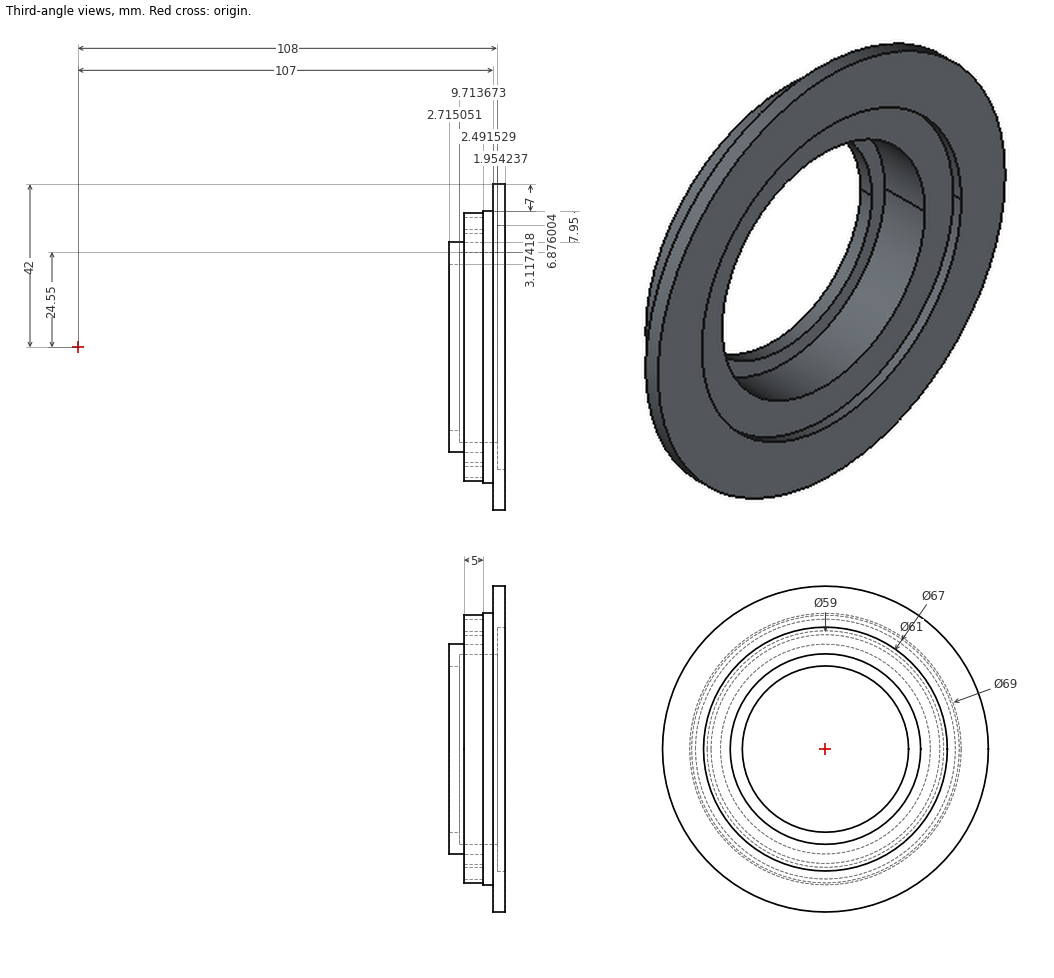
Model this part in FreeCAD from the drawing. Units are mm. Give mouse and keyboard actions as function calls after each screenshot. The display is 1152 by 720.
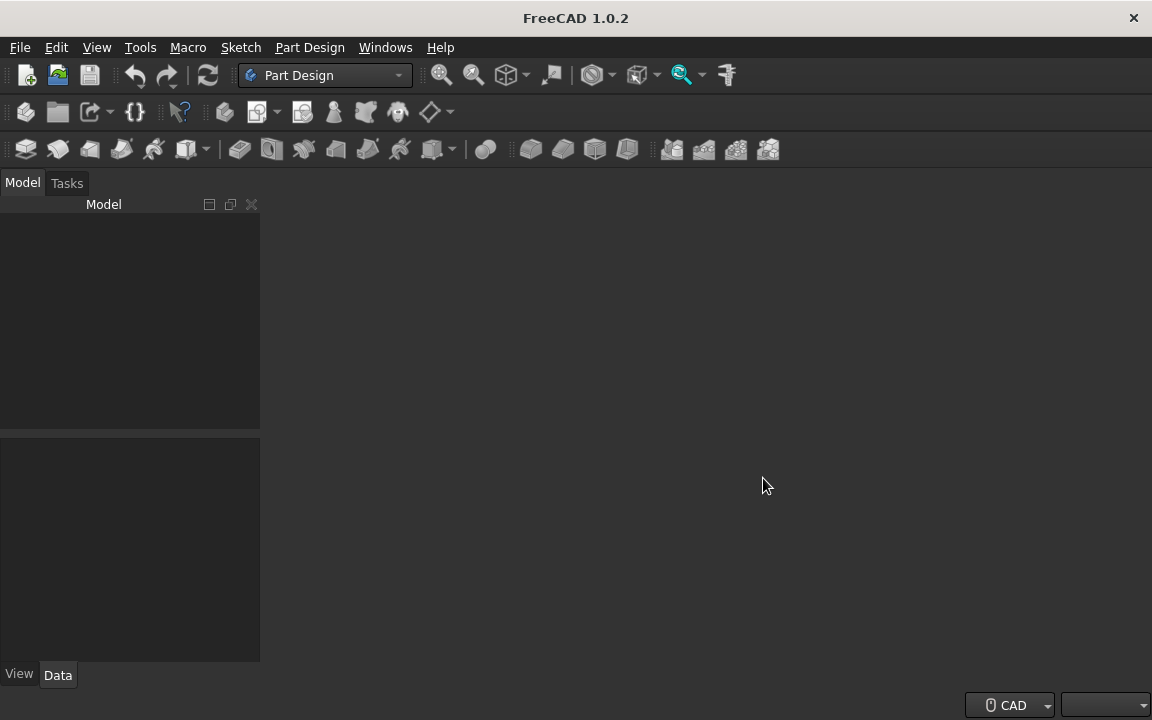
click(26, 76)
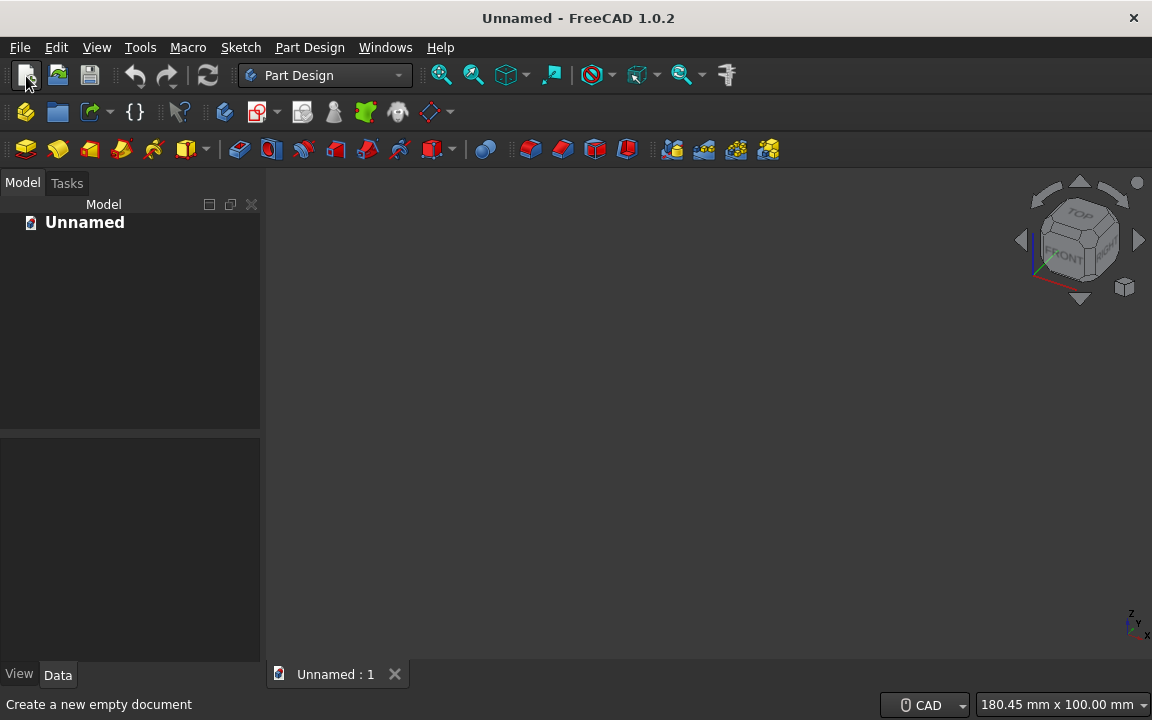
click(258, 112)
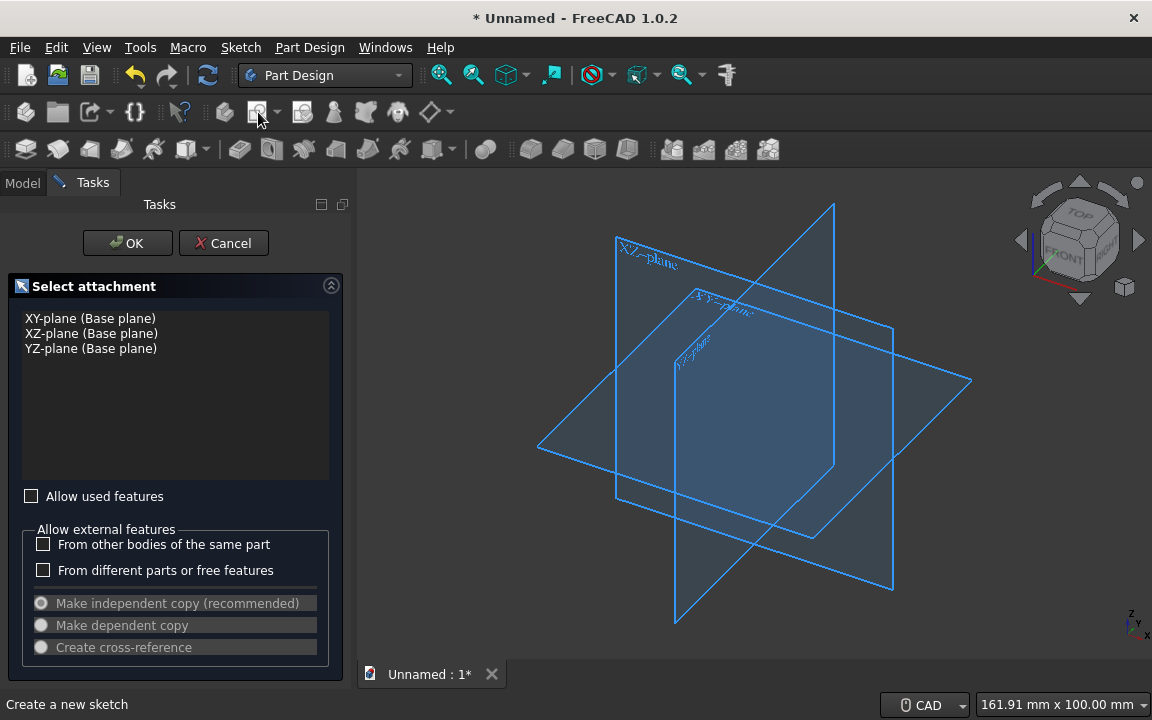
click(82, 318)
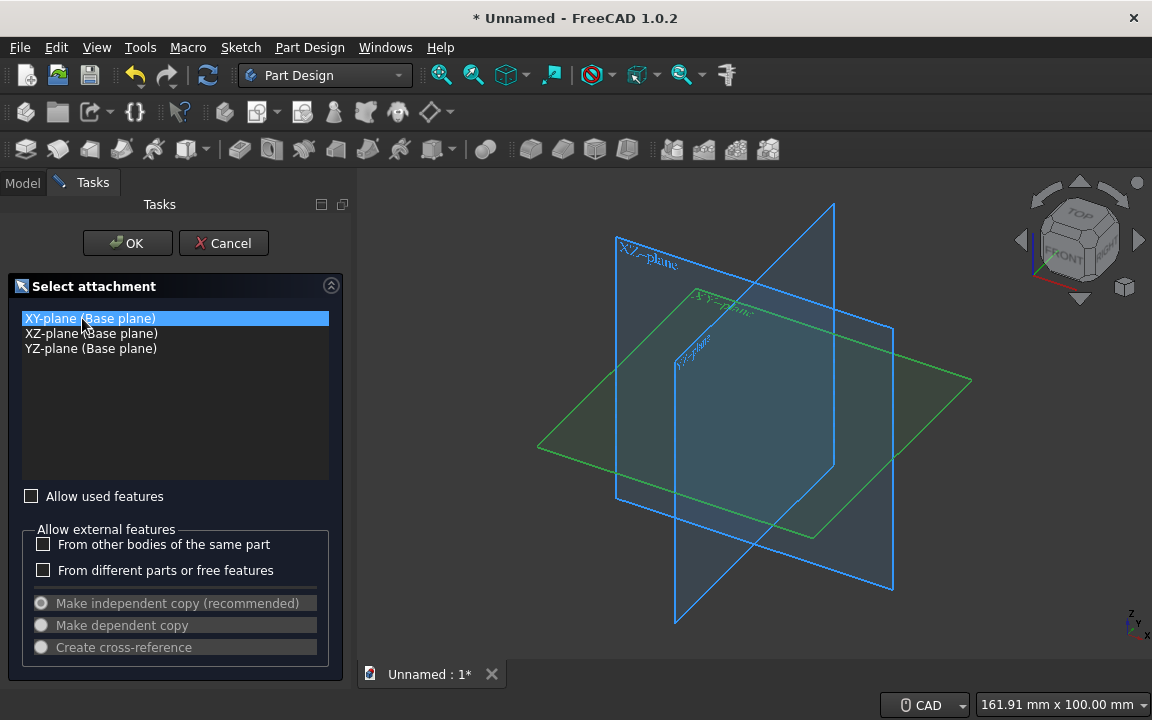
click(128, 243)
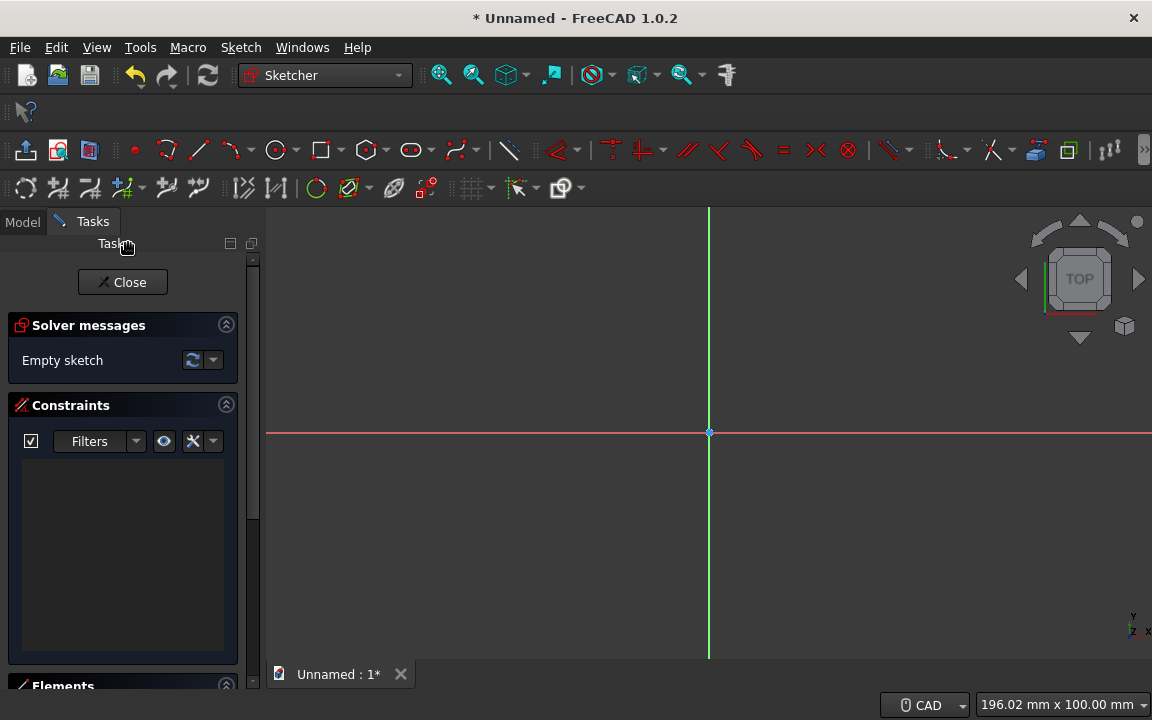
scroll(640, 433, down, 5)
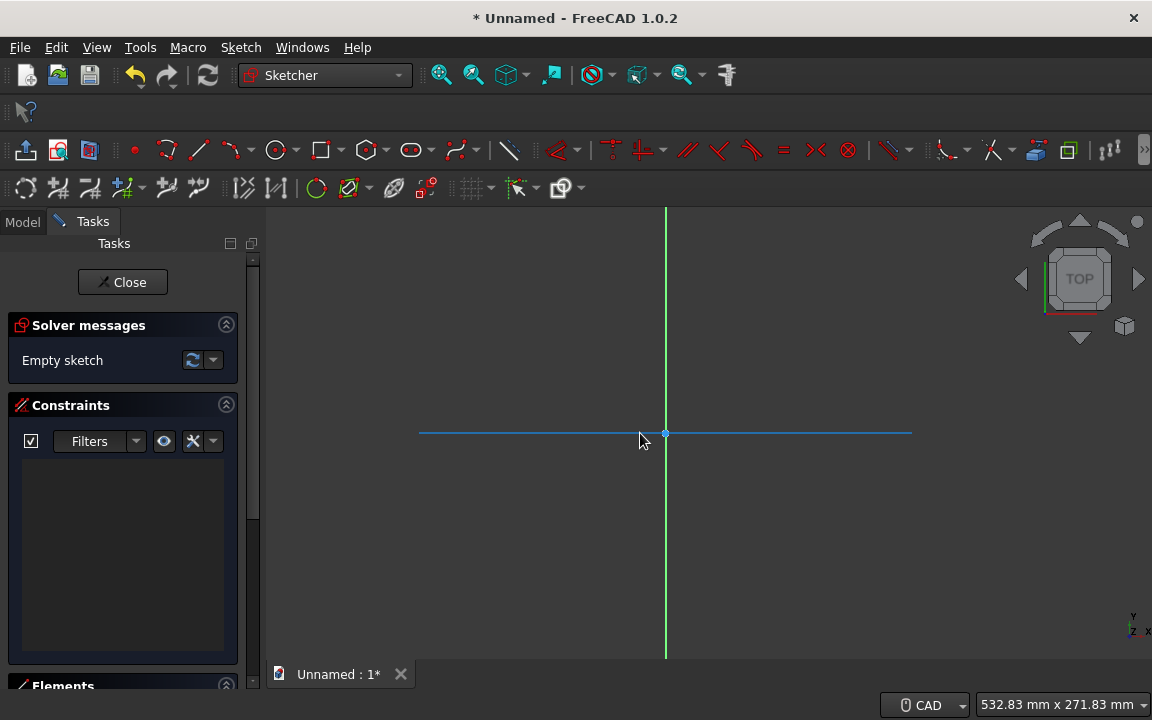
scroll(861, 374, up, 11)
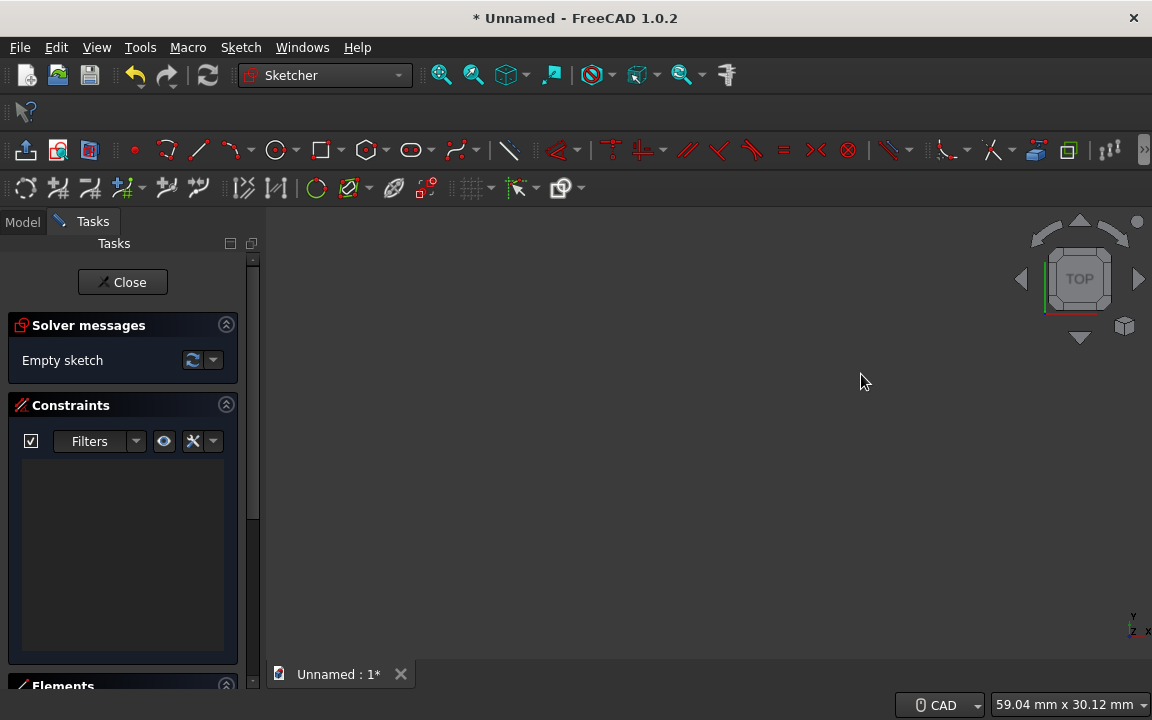
click(168, 150)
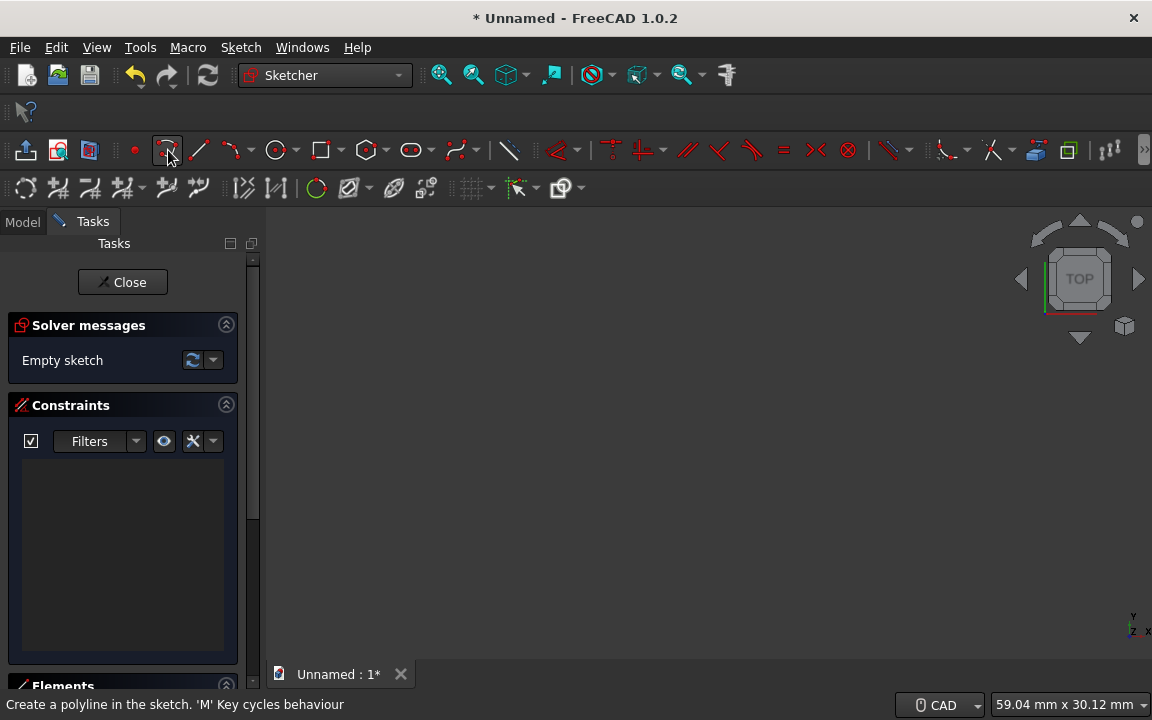
click(527, 585)
click(568, 585)
click(568, 538)
click(713, 538)
click(713, 435)
click(743, 435)
click(743, 276)
click(698, 276)
click(698, 381)
click(661, 381)
click(661, 500)
click(527, 500)
click(527, 586)
key(Escape)
key(Escape)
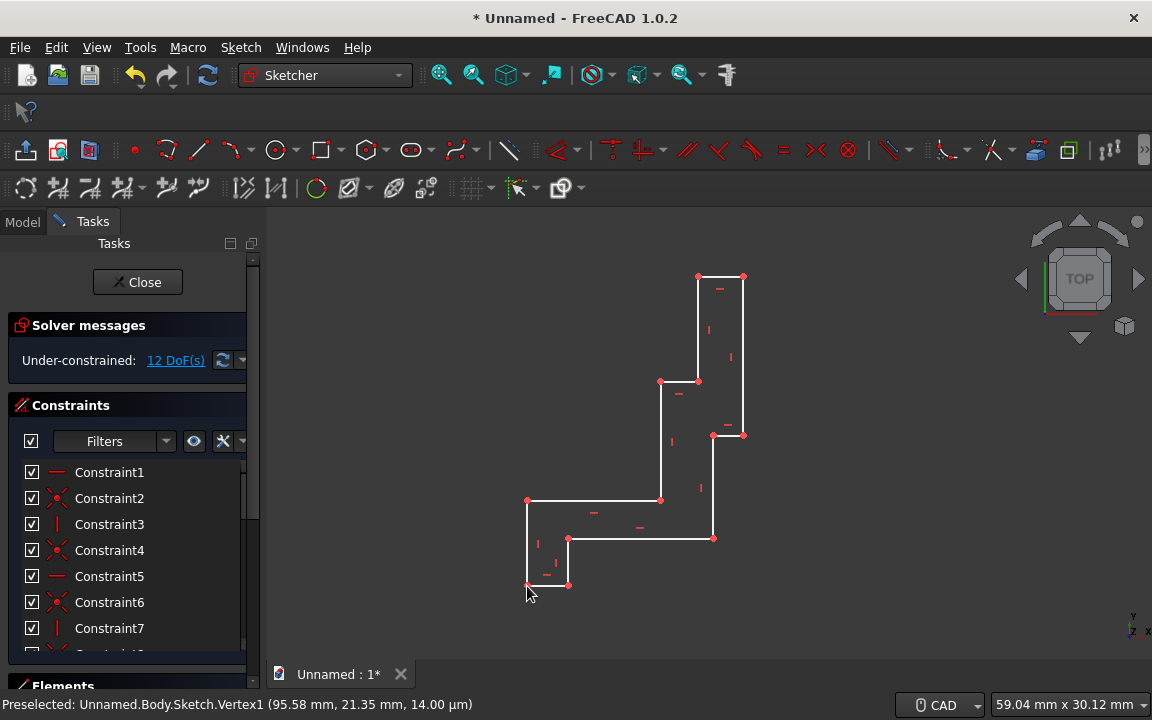
click(556, 150)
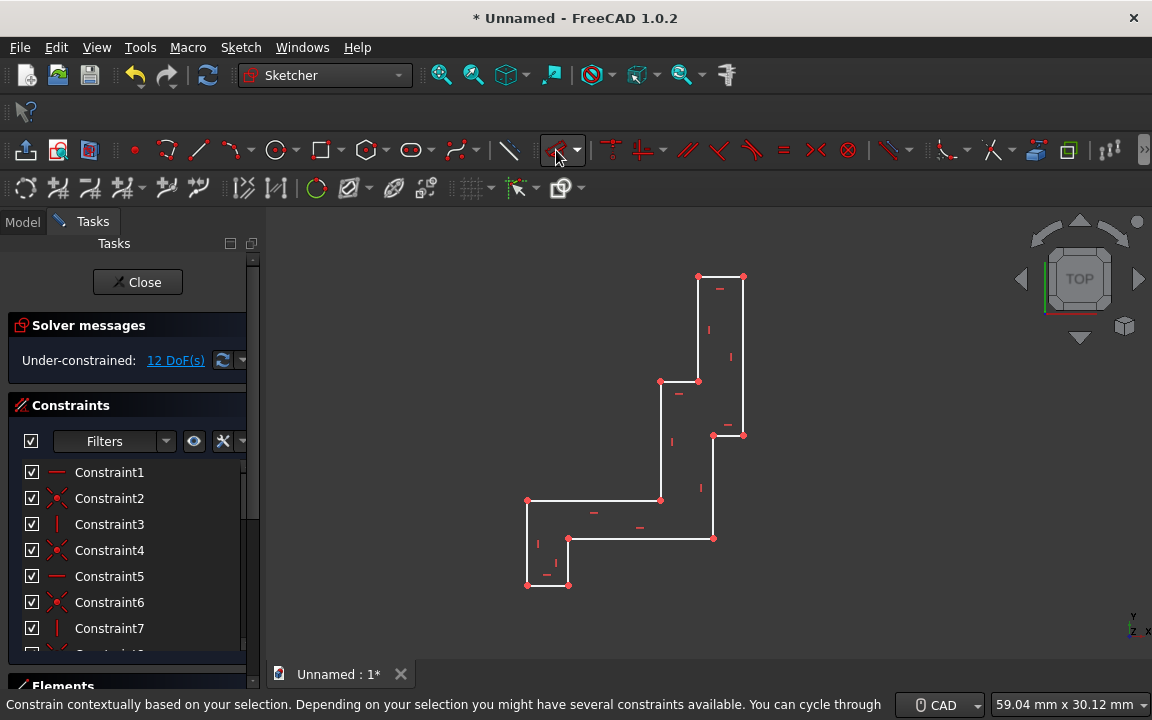
click(698, 309)
click(664, 330)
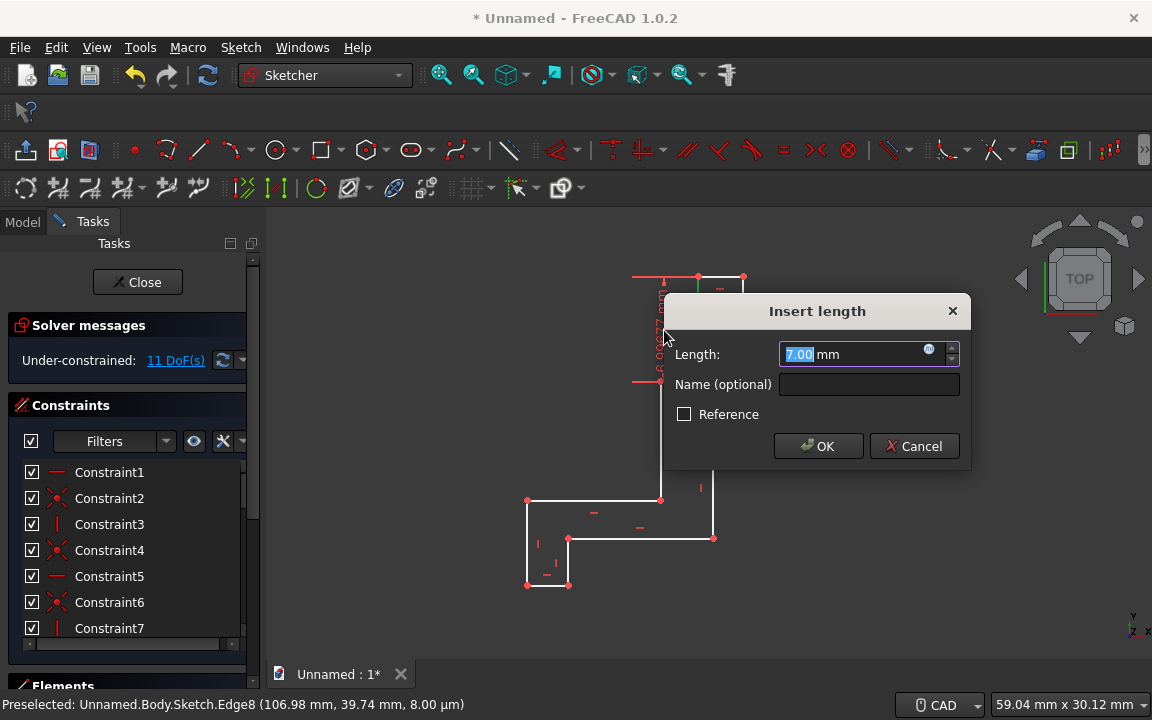
text(7)
key(Return)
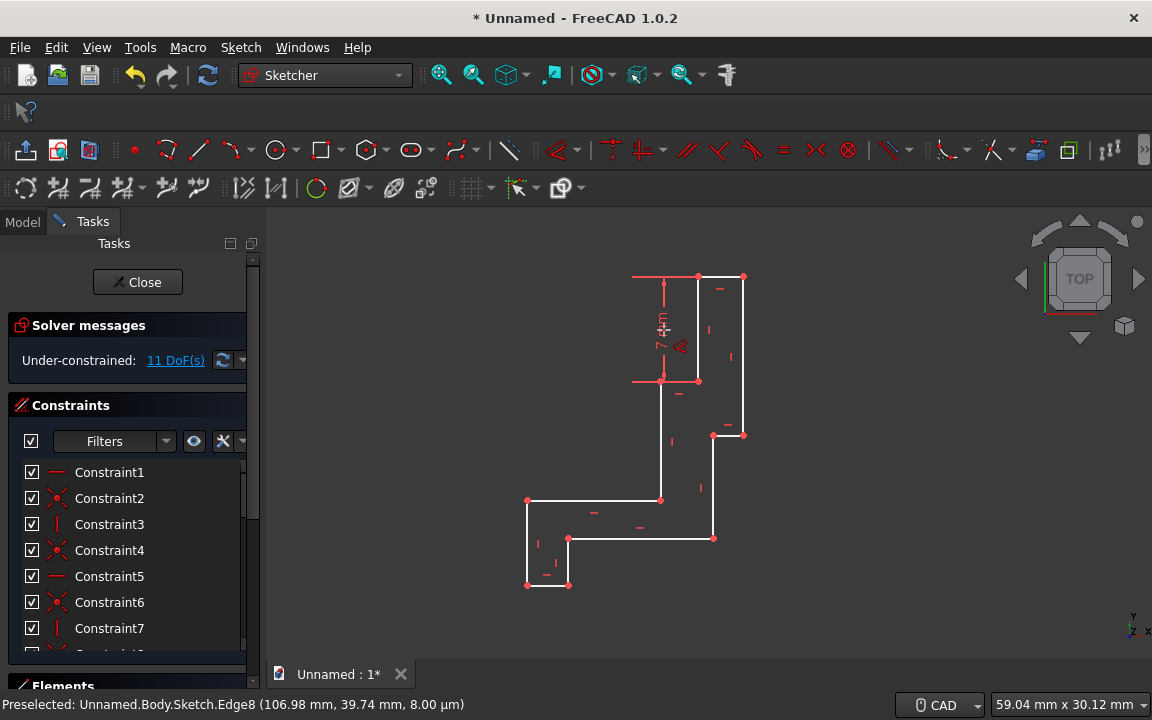
click(743, 277)
click(777, 454)